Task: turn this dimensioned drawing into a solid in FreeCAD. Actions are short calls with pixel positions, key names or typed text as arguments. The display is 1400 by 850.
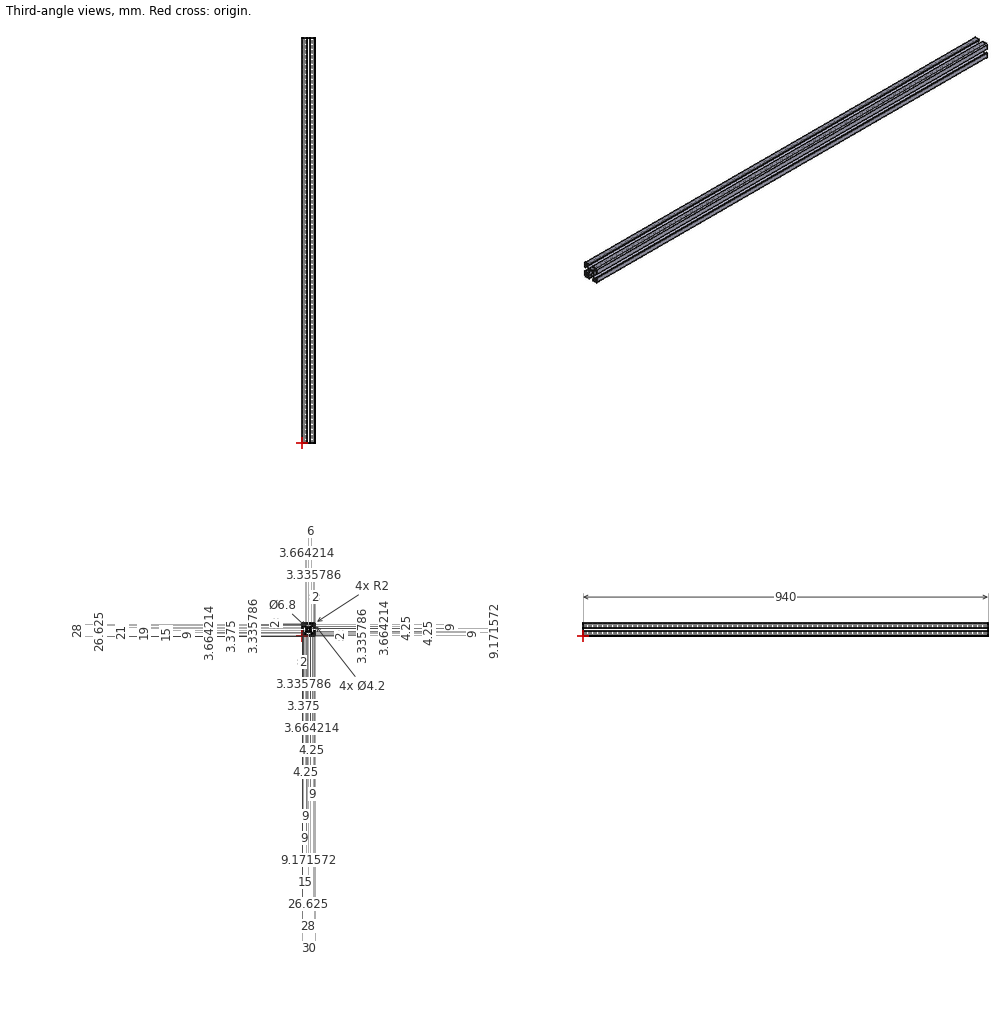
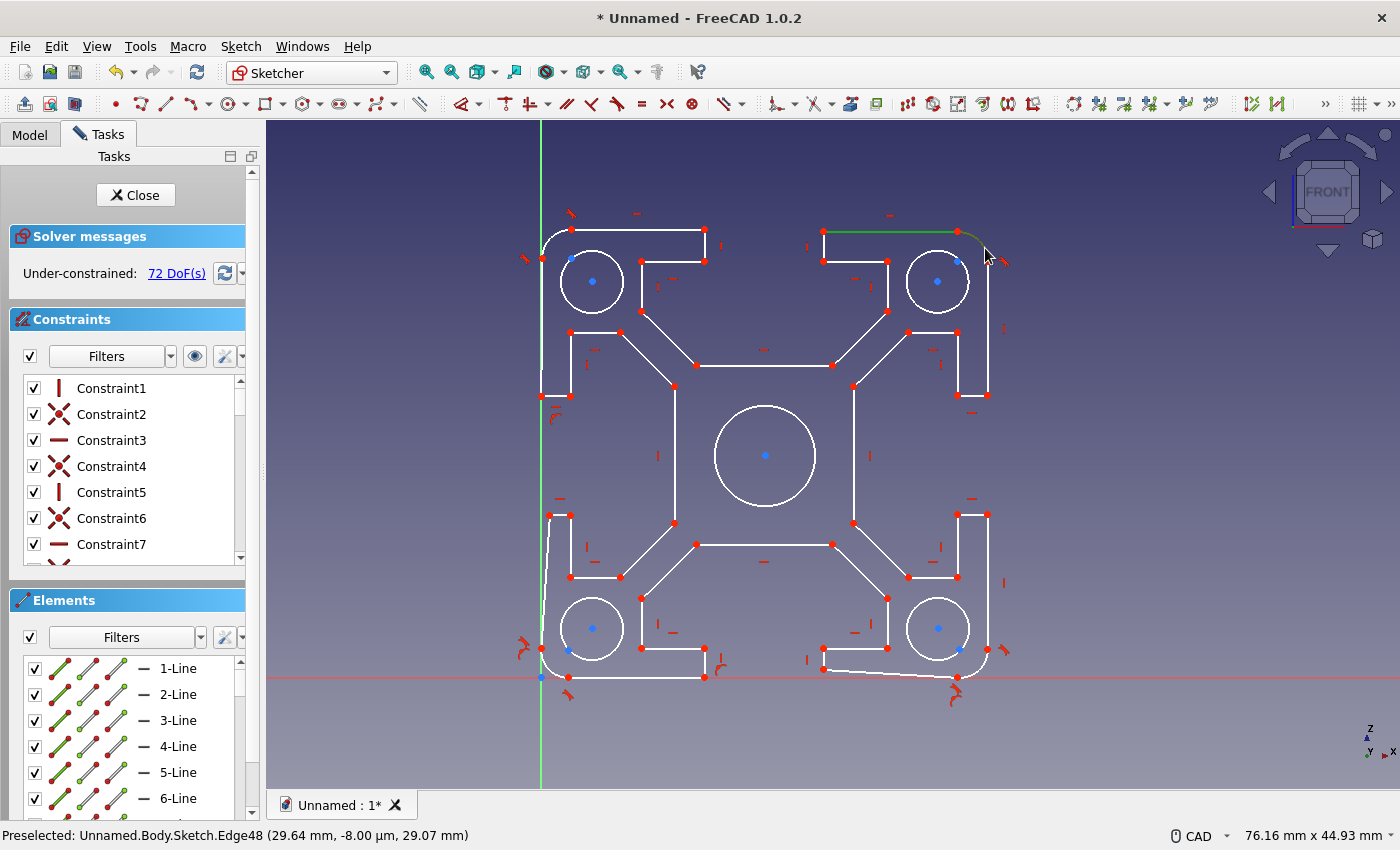
key(t)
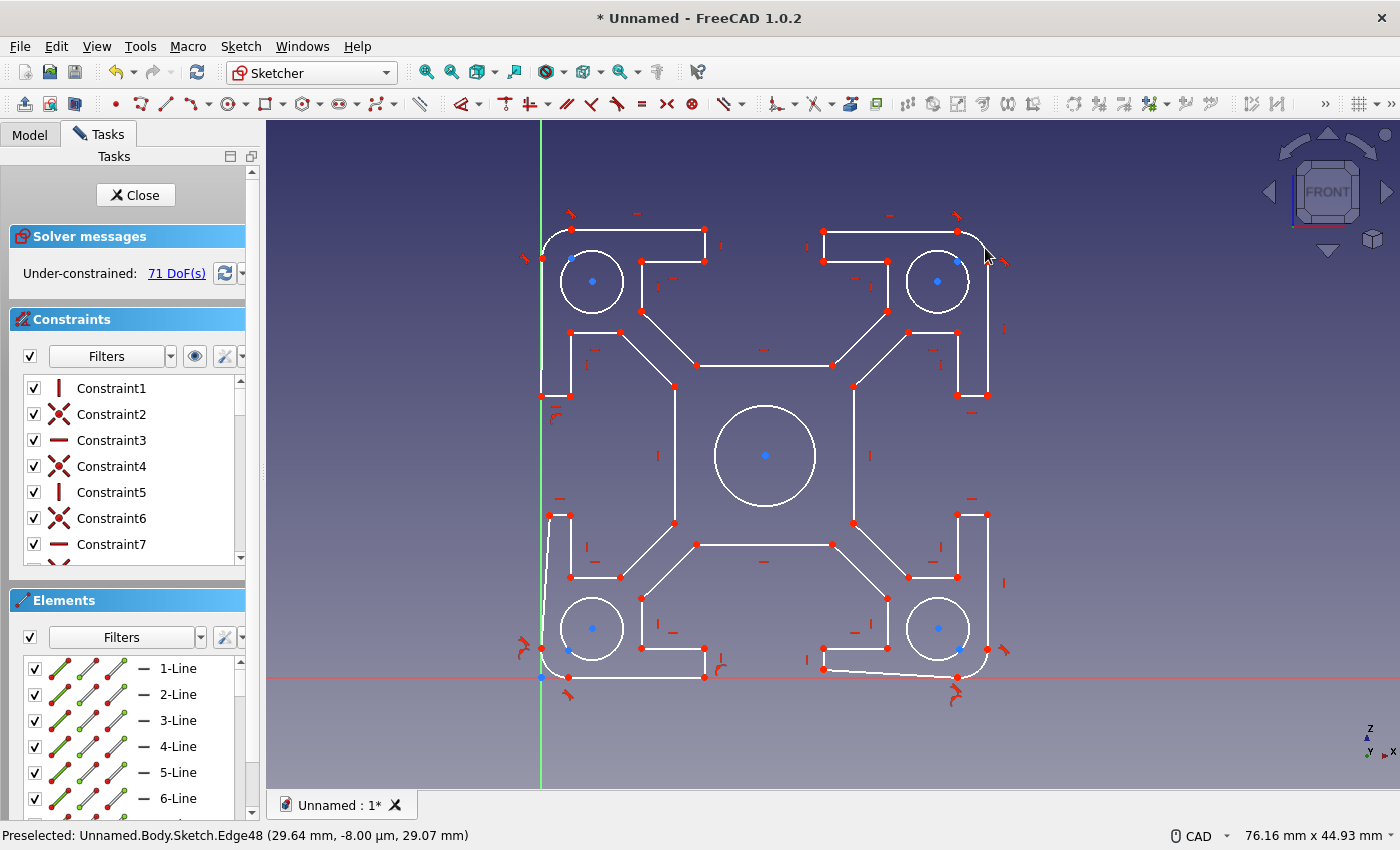
click(918, 676)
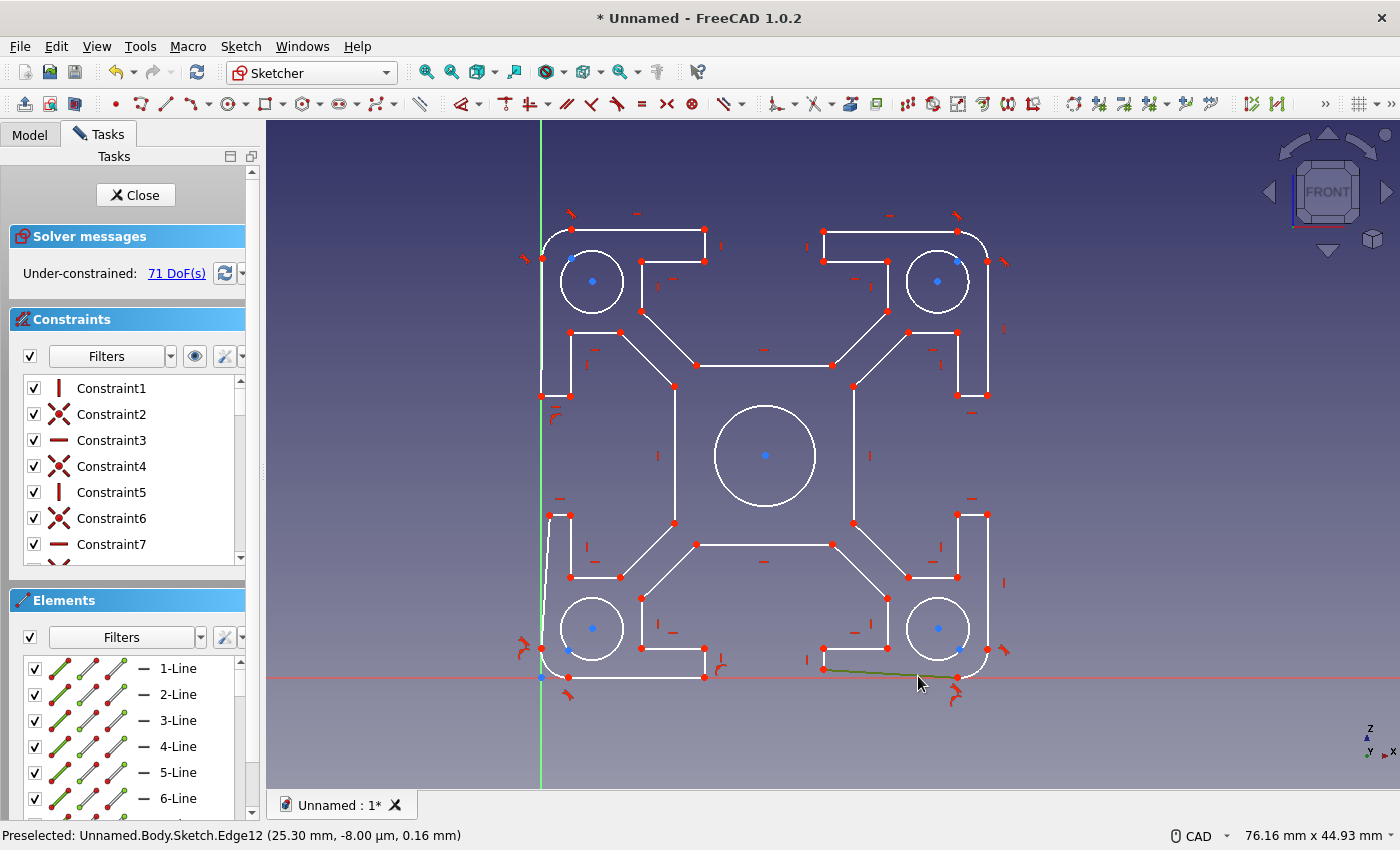
click(548, 104)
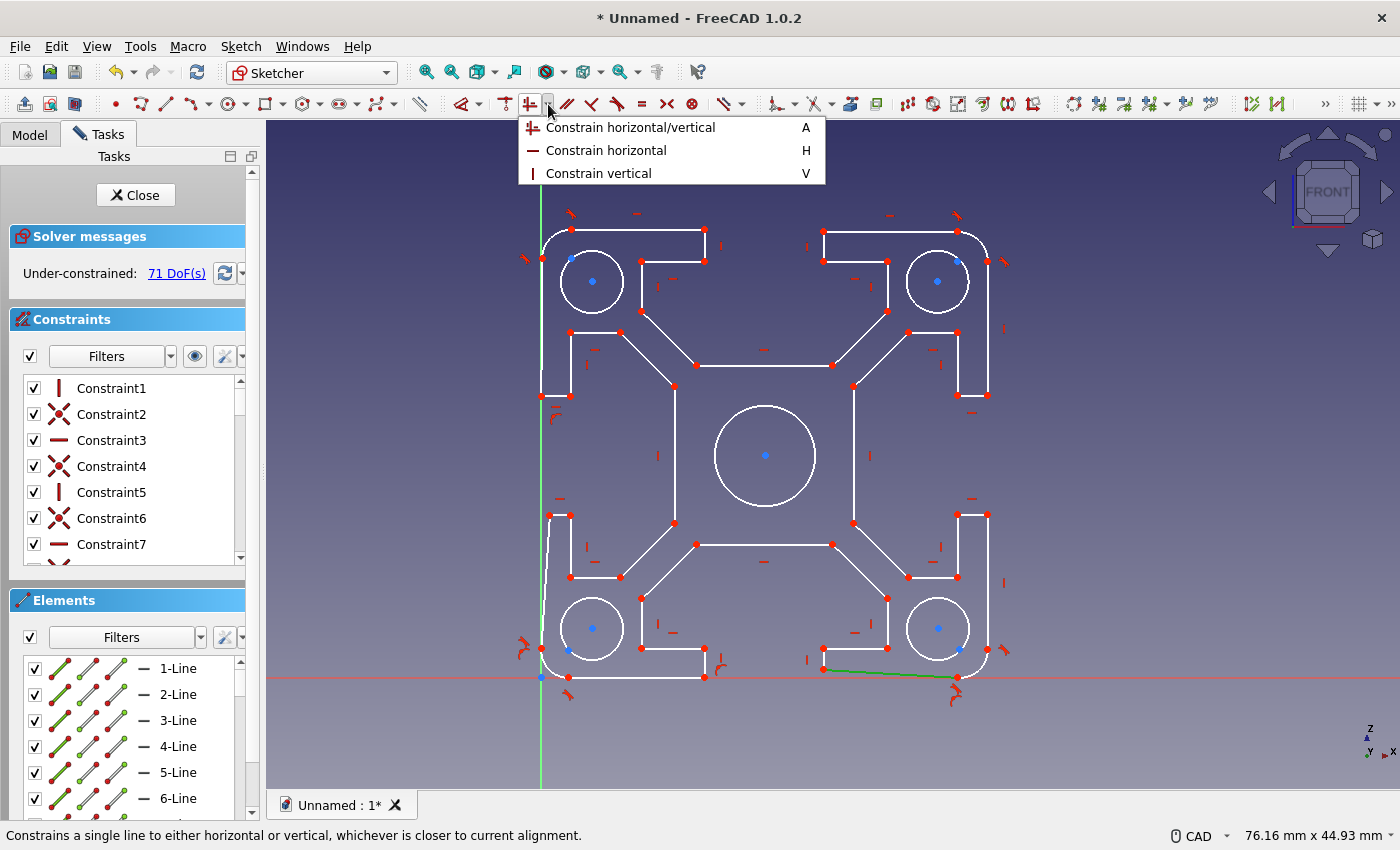
click(672, 150)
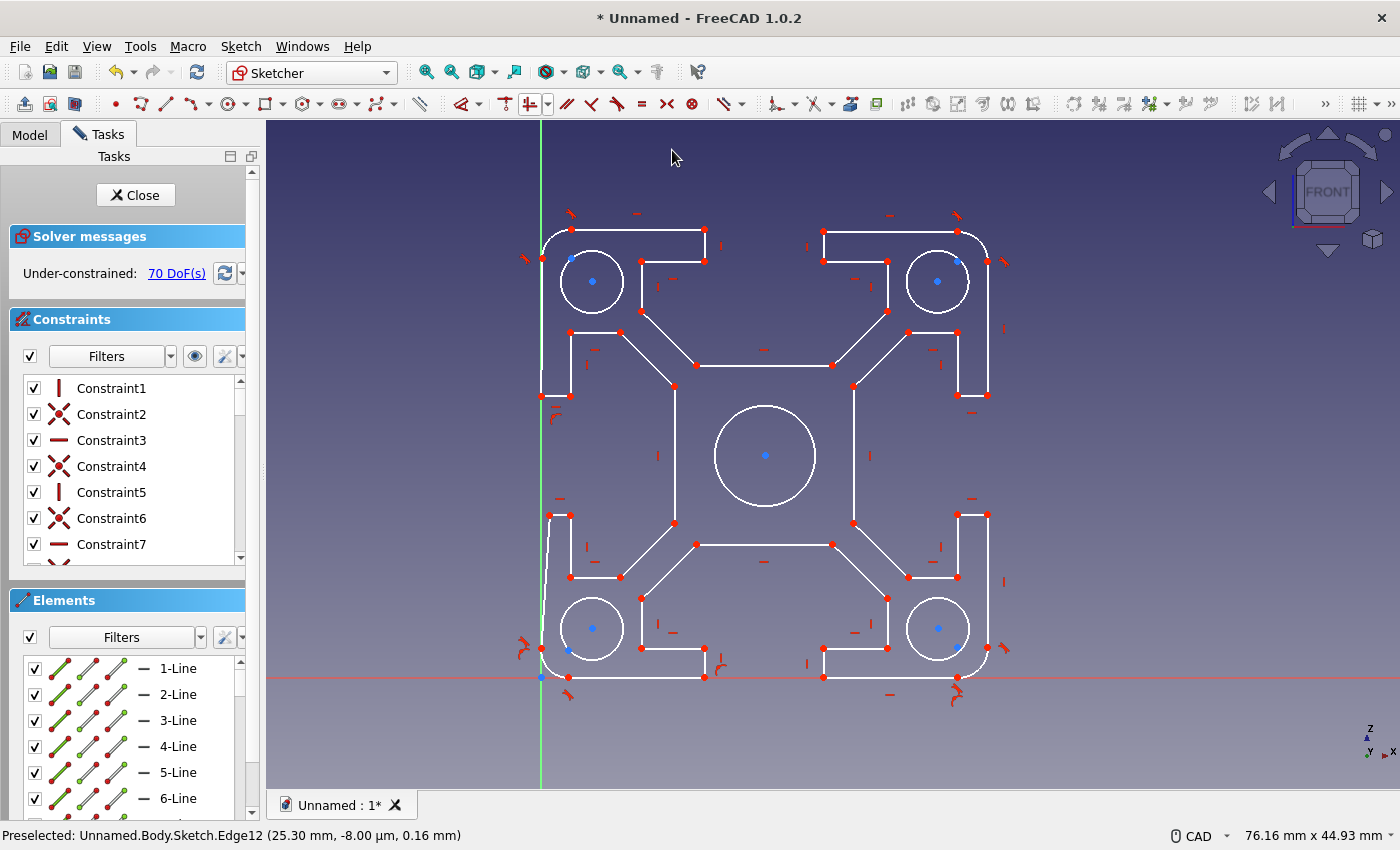
click(664, 678)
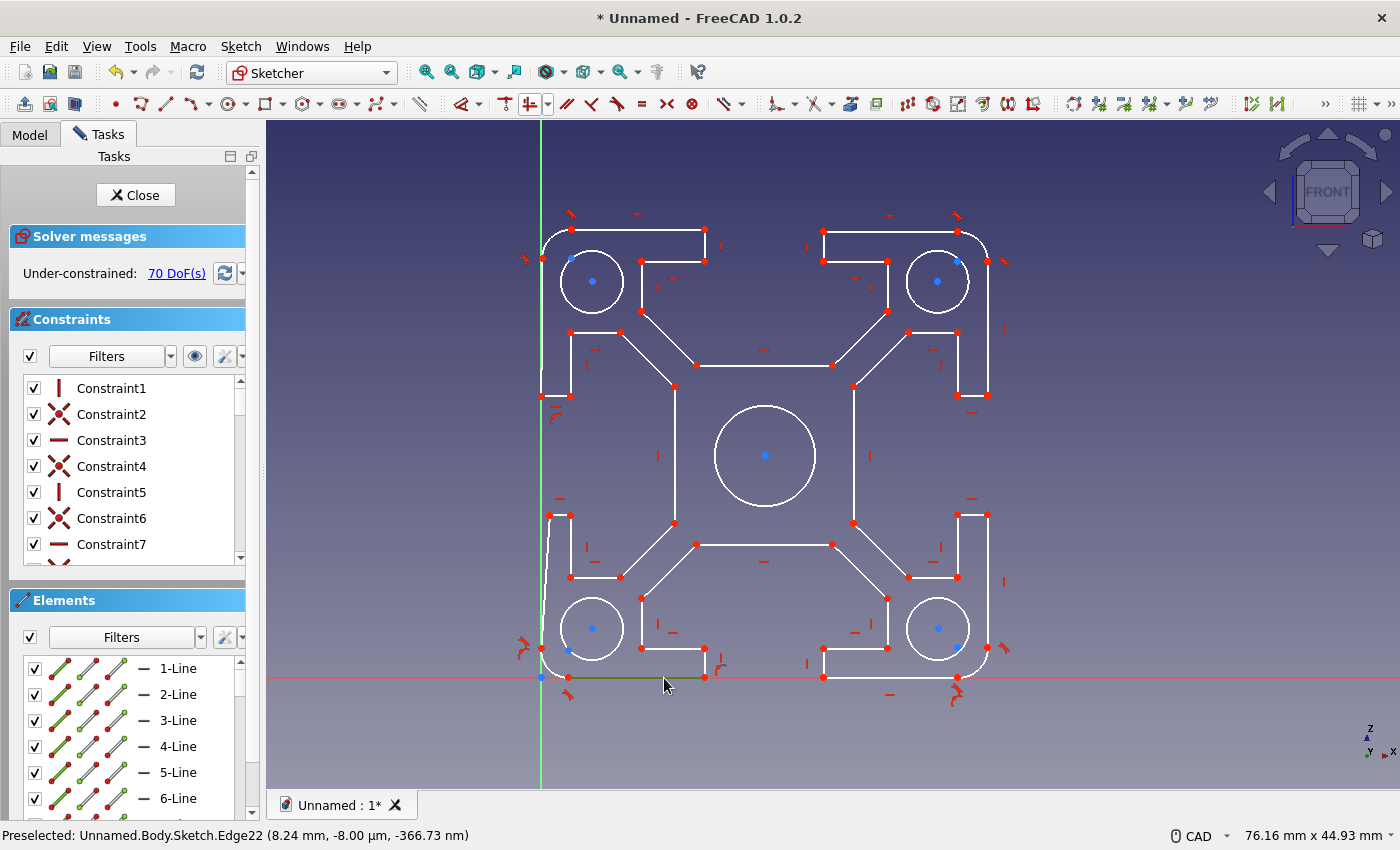
key(h)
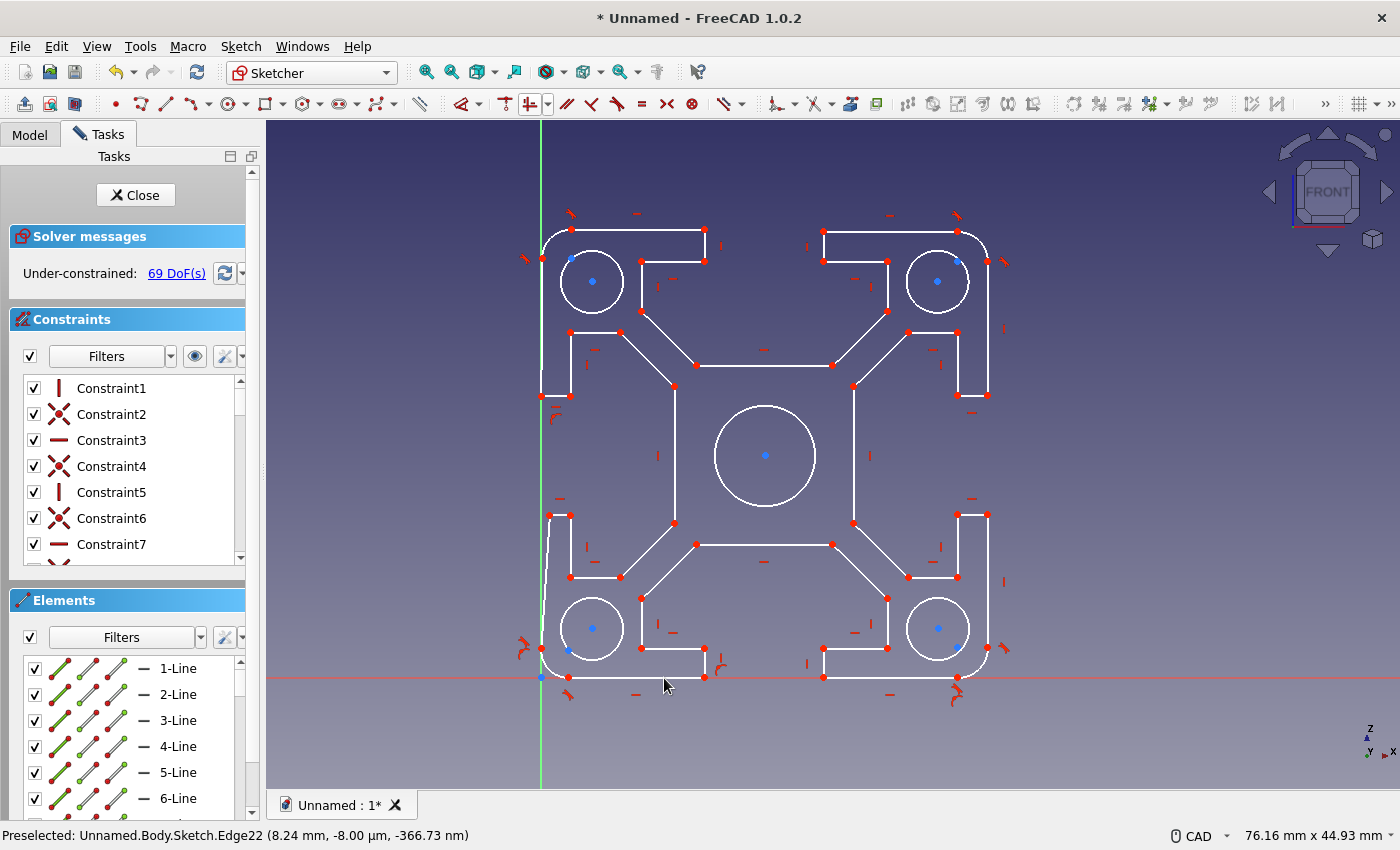
click(544, 609)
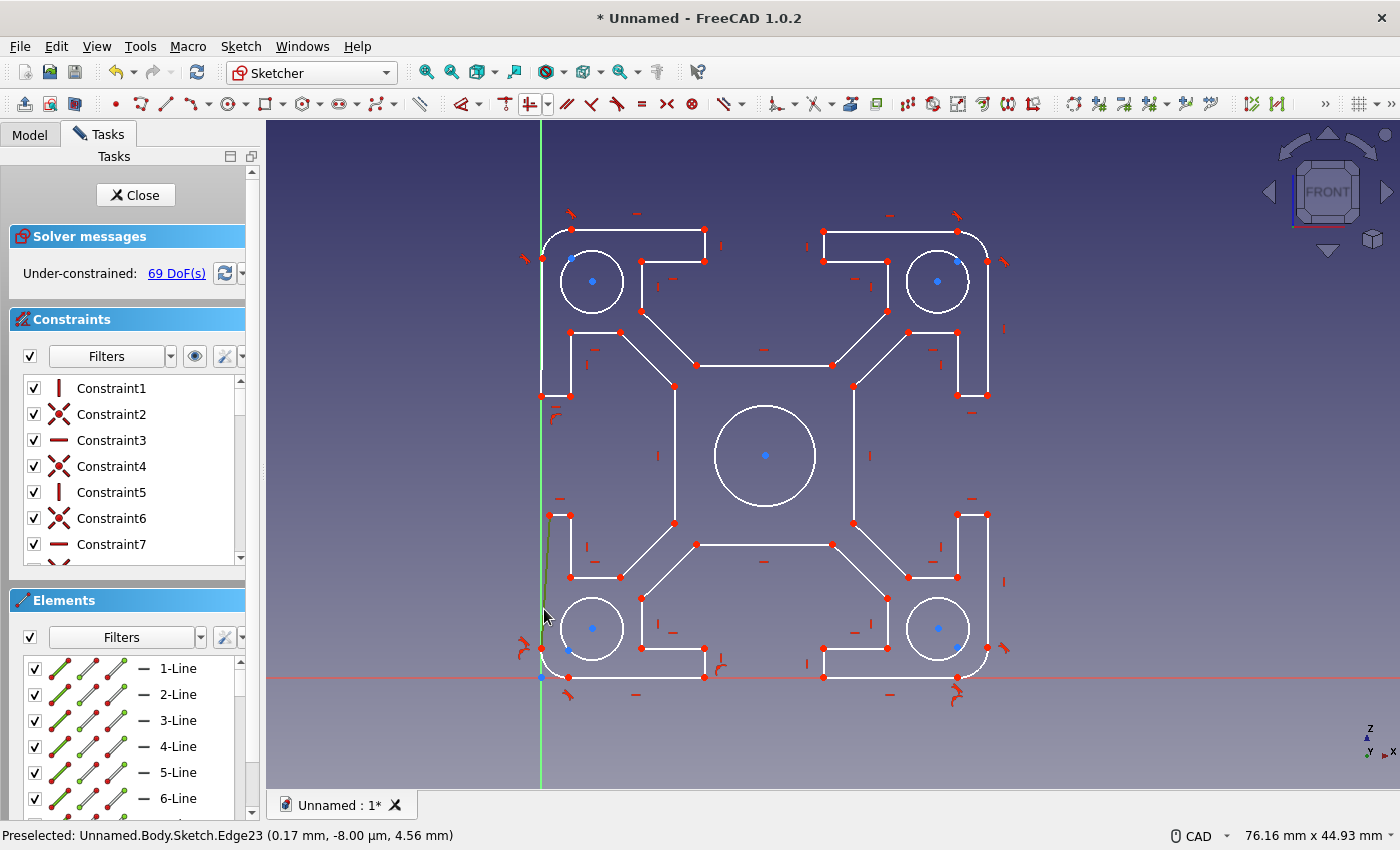
click(548, 104)